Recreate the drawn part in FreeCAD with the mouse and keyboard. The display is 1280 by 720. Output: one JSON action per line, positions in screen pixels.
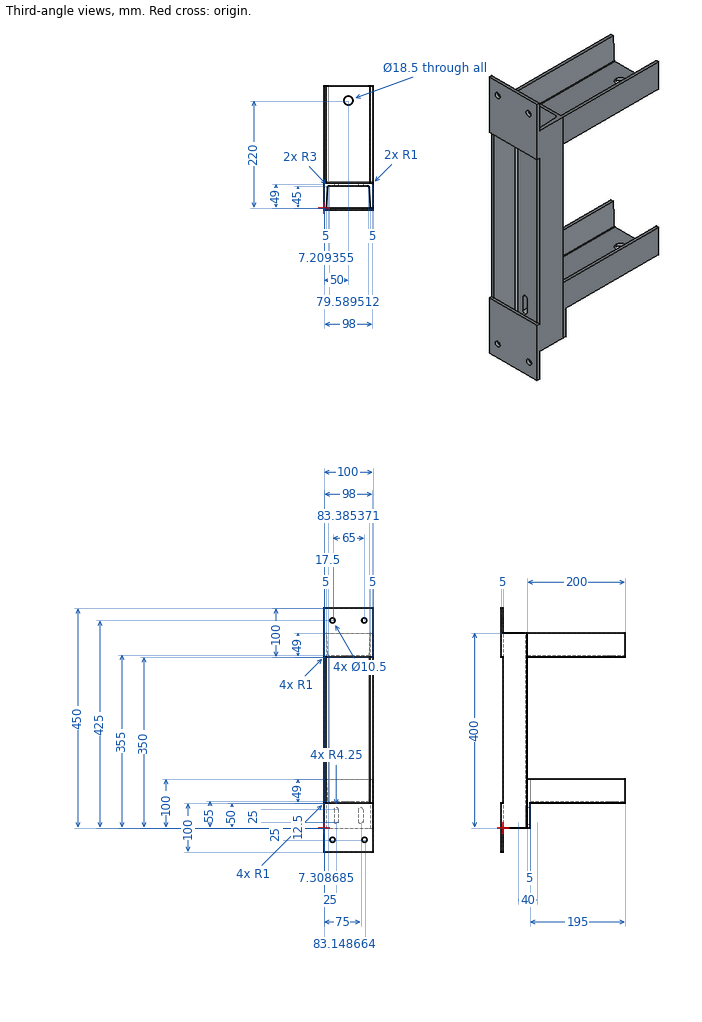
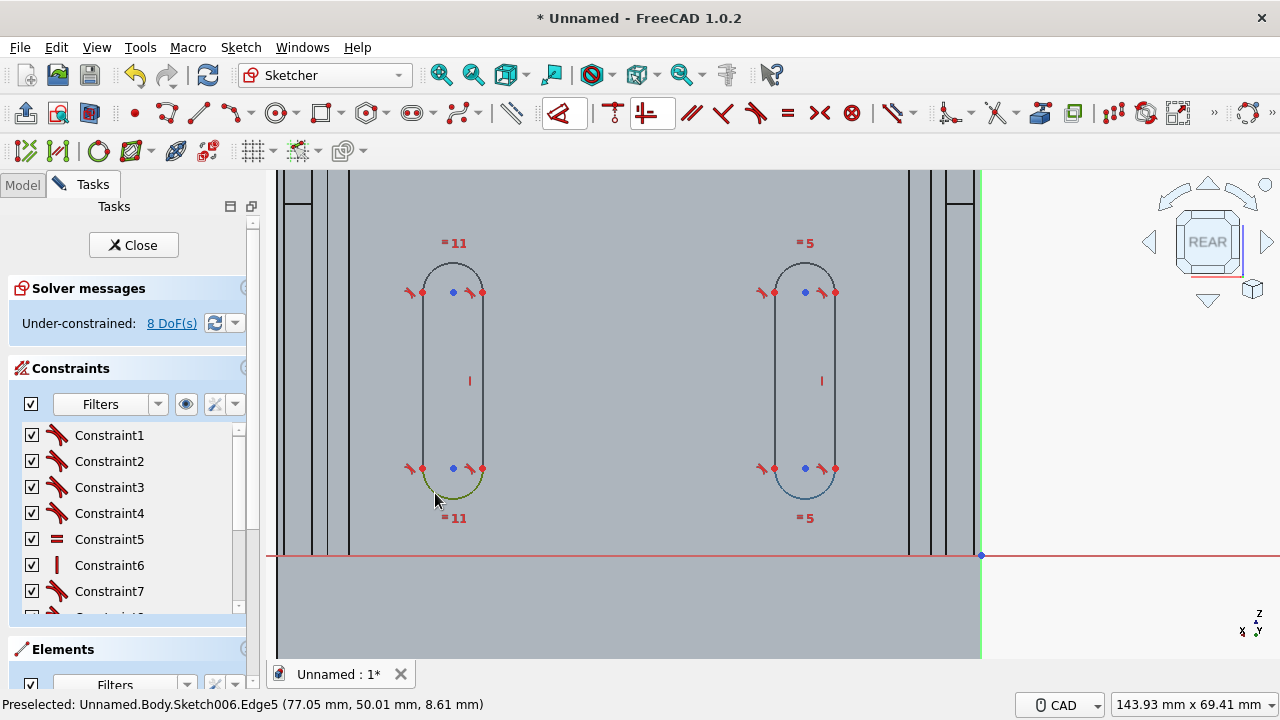
{"action": "left_click", "coordinate": [788, 114]}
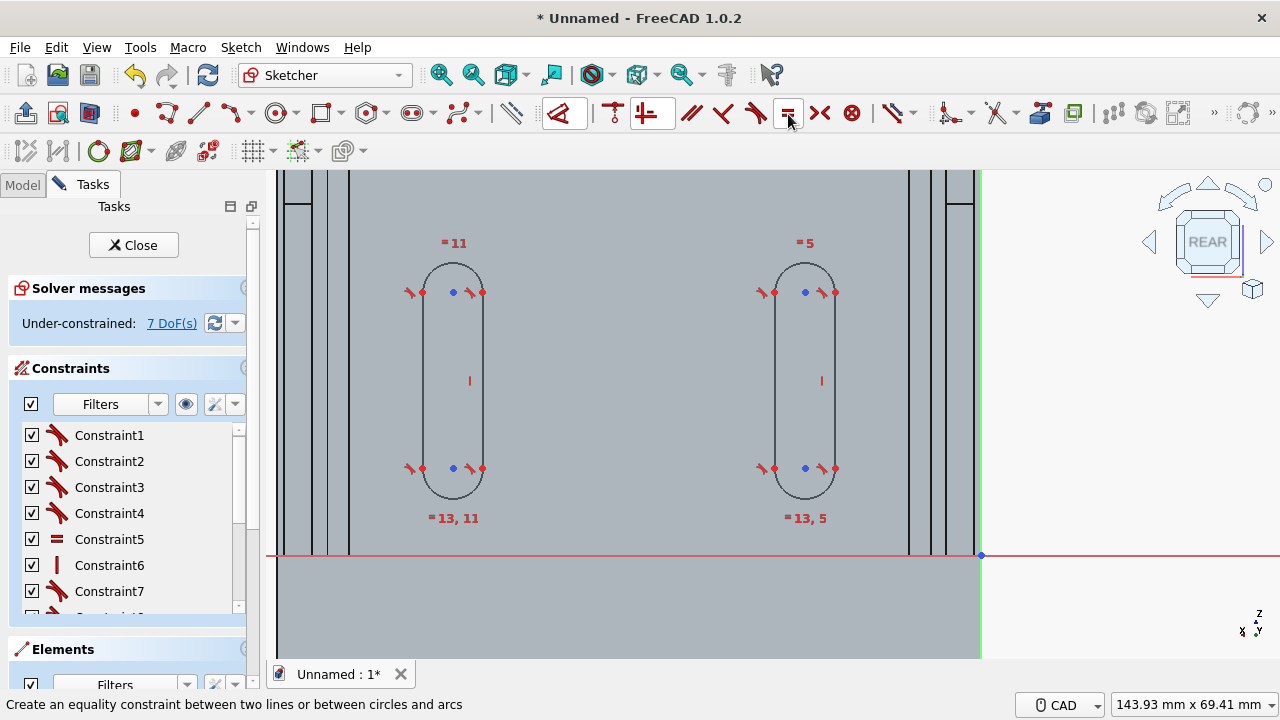
{"action": "scroll", "coordinate": [787, 493], "scroll_direction": "up", "scroll_amount": 2}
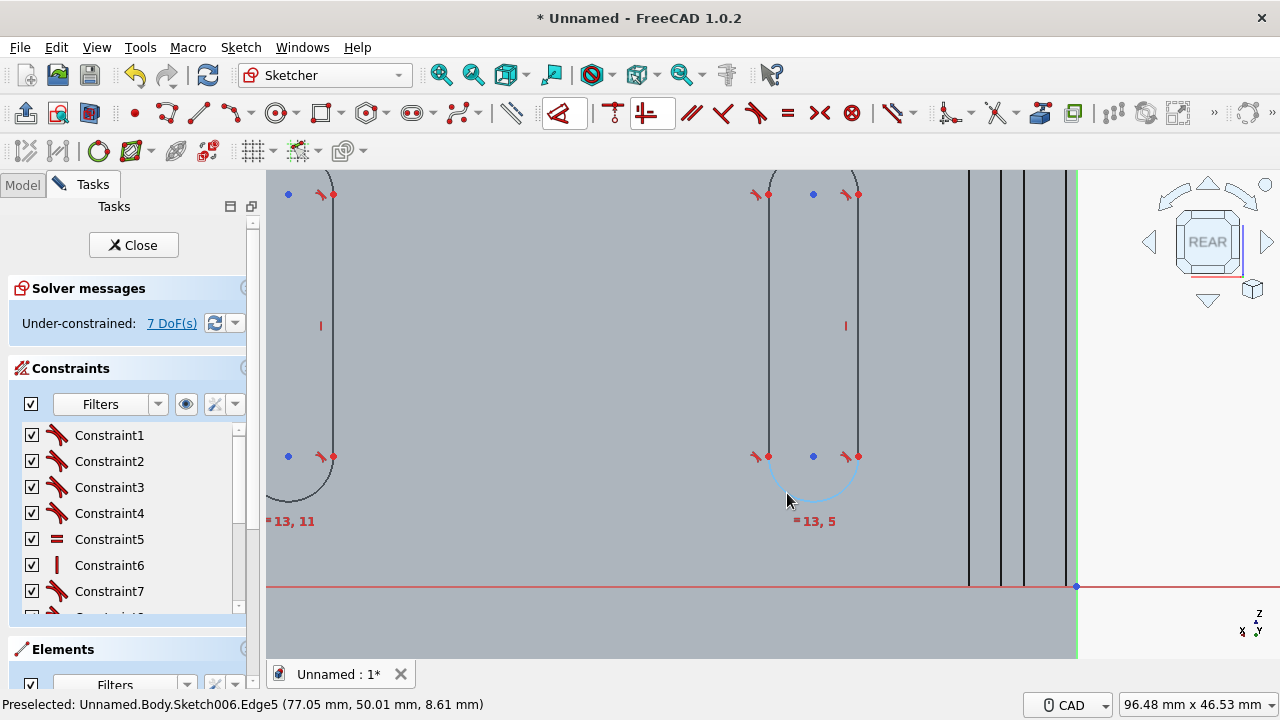
{"action": "left_click", "coordinate": [787, 493]}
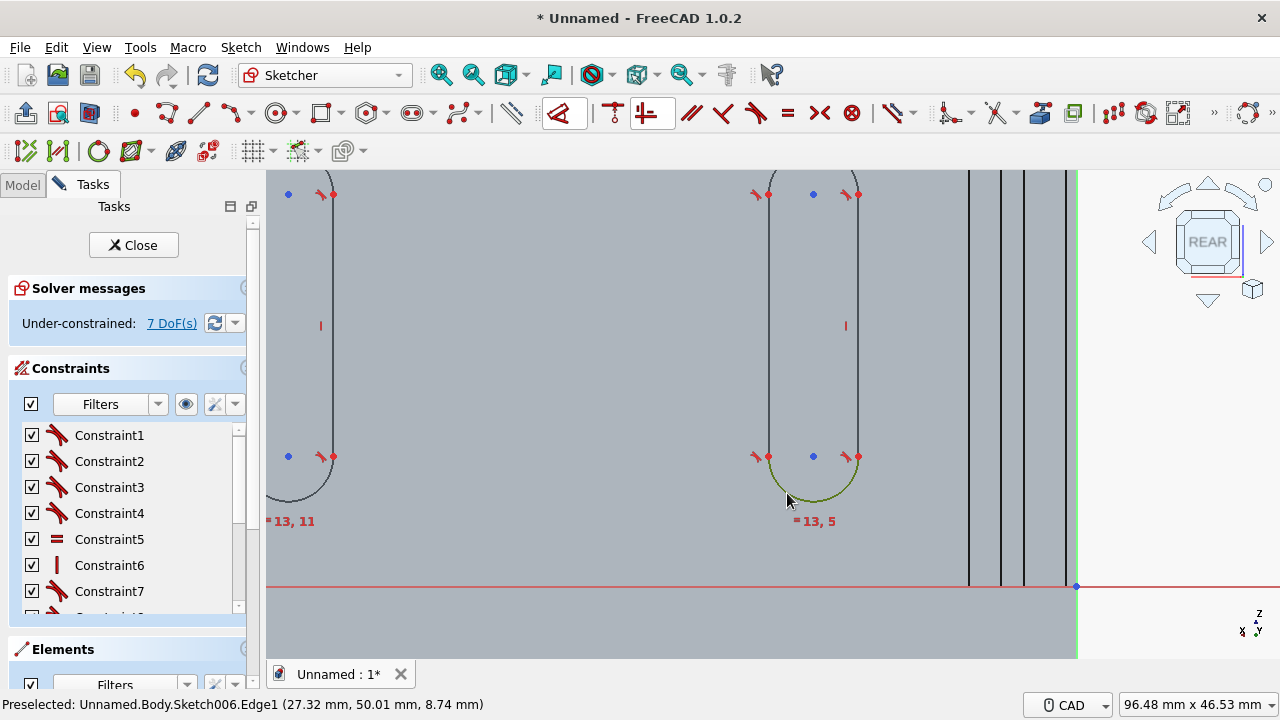
{"action": "key", "text": "k r"}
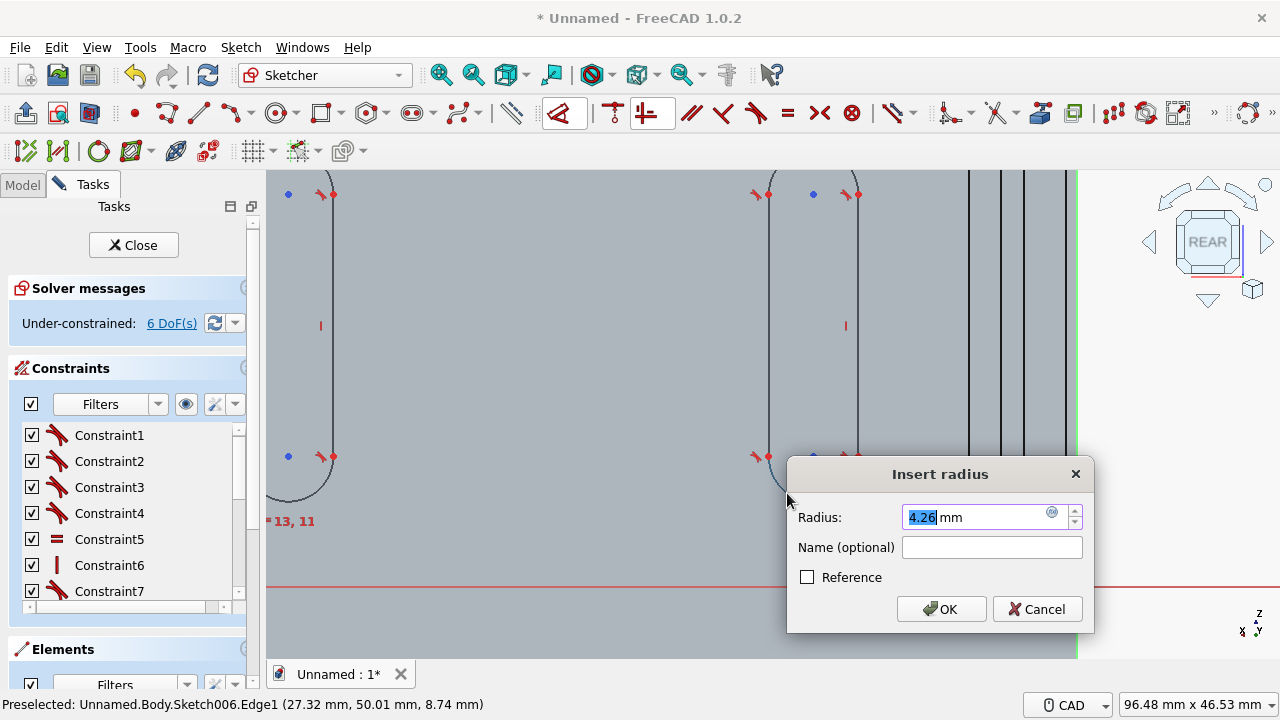
{"action": "type", "text": "4.25"}
{"action": "key", "text": "Return"}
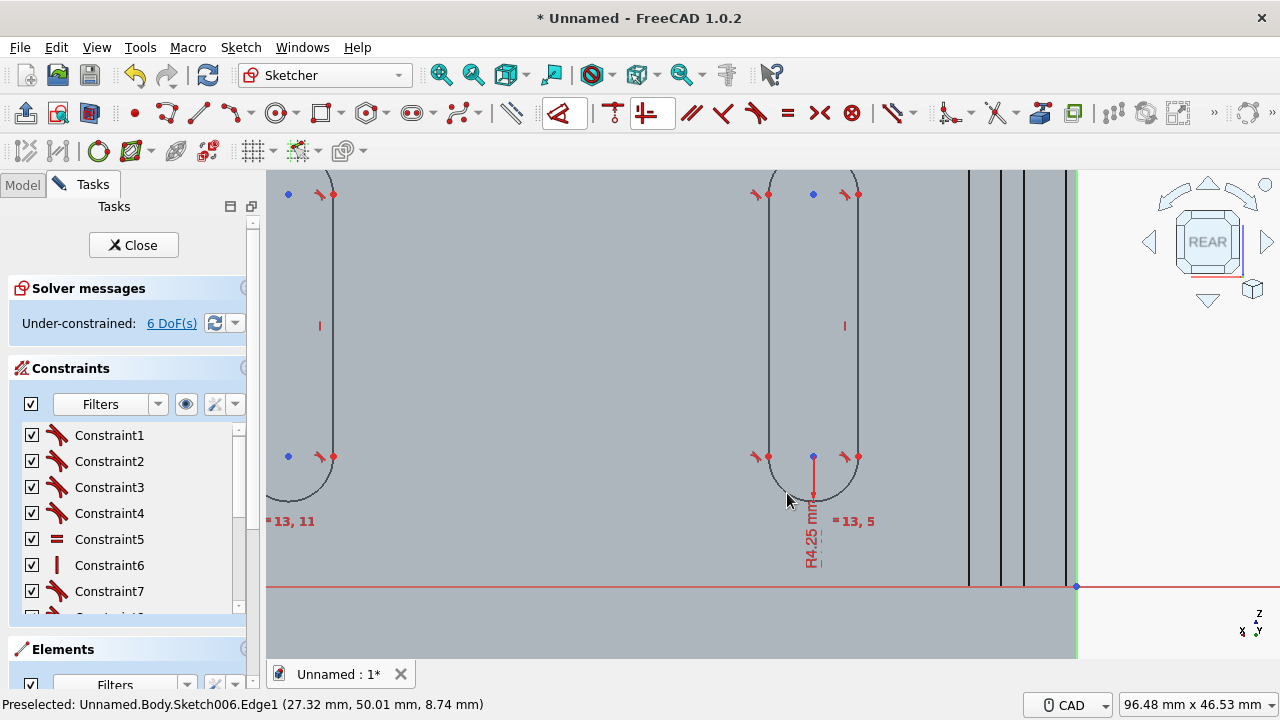
{"action": "left_click", "coordinate": [769, 378]}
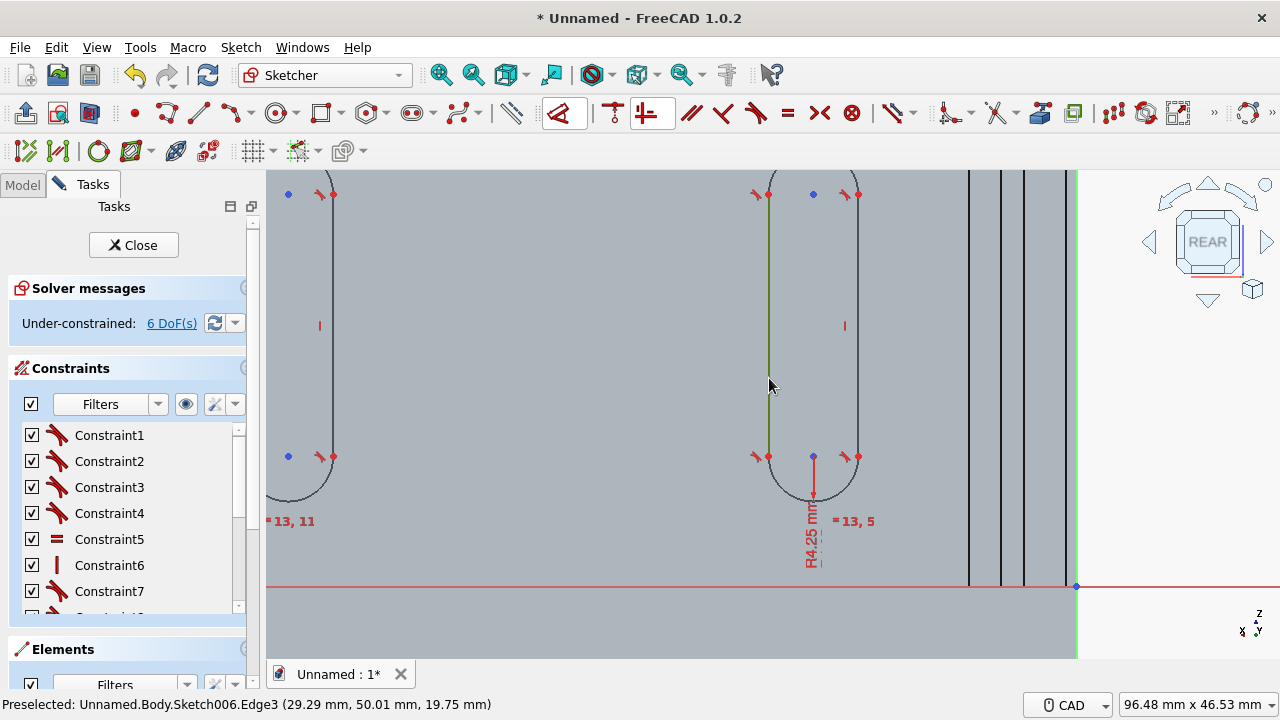
{"action": "left_click", "coordinate": [582, 114]}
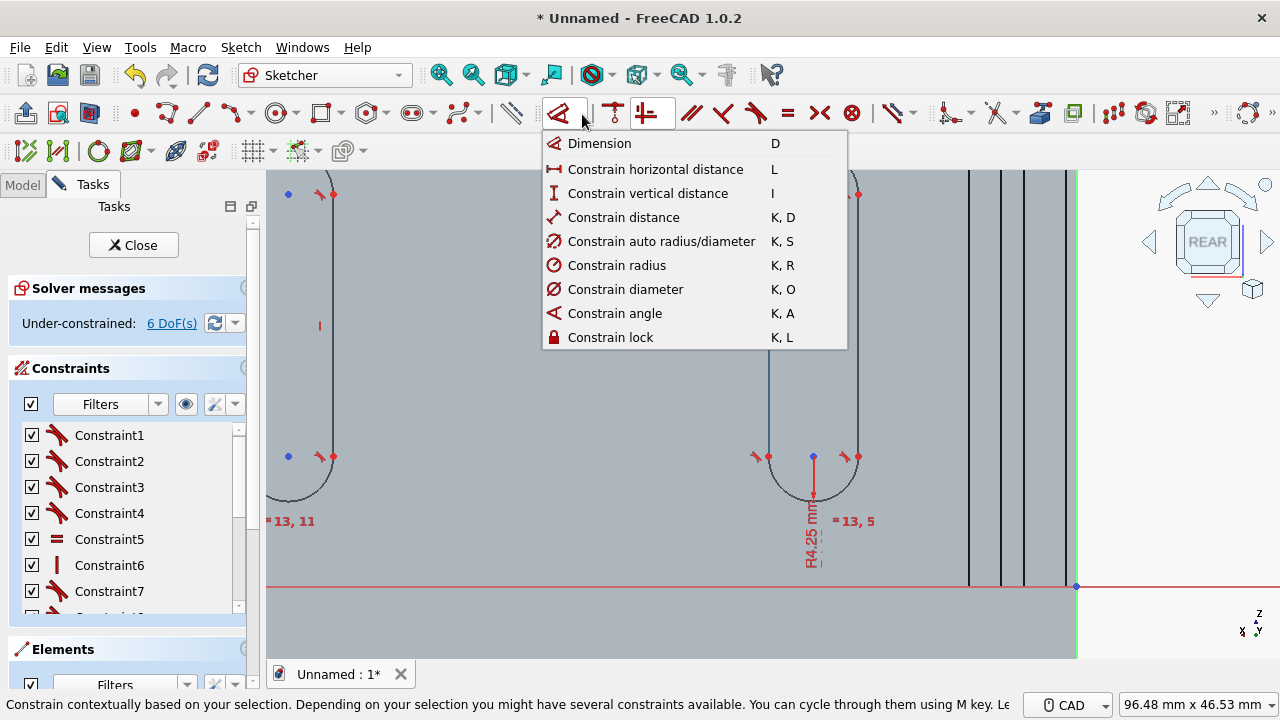
{"action": "left_click", "coordinate": [695, 193]}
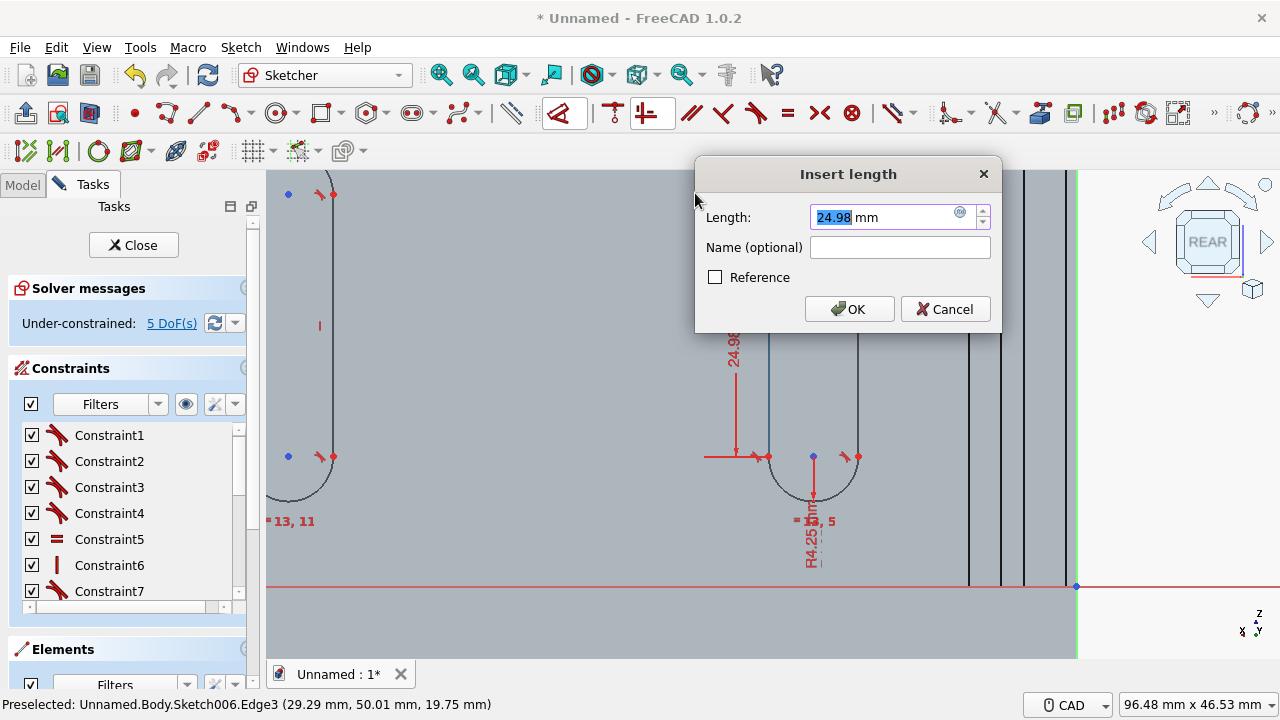
{"action": "type", "text": "25"}
{"action": "key", "text": "Return"}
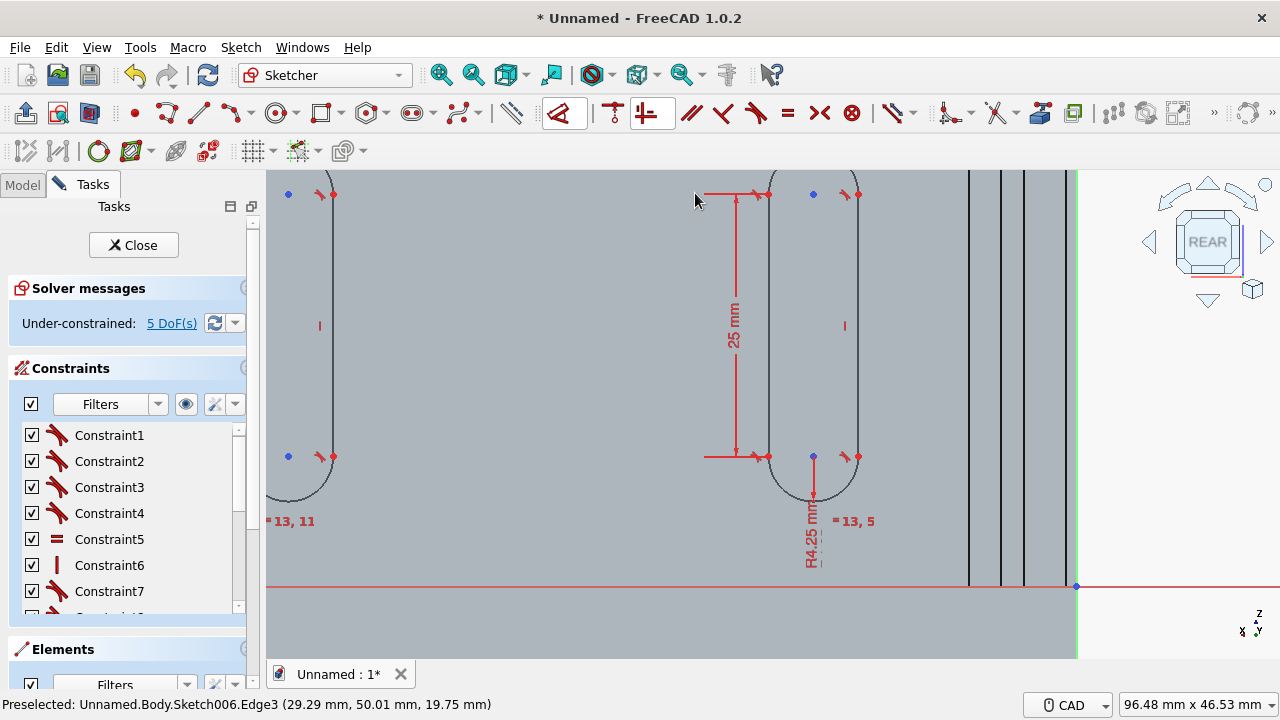
{"action": "scroll", "coordinate": [794, 511], "scroll_direction": "down", "scroll_amount": 2}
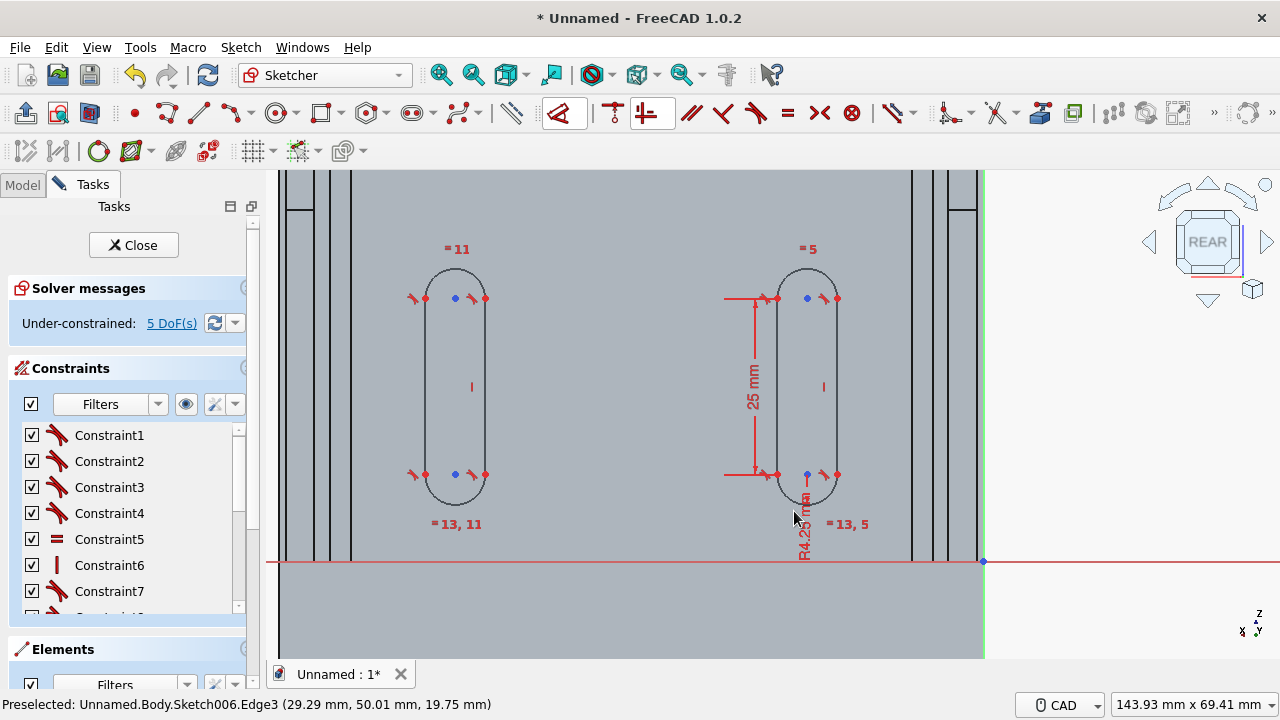
{"action": "left_click", "coordinate": [425, 422]}